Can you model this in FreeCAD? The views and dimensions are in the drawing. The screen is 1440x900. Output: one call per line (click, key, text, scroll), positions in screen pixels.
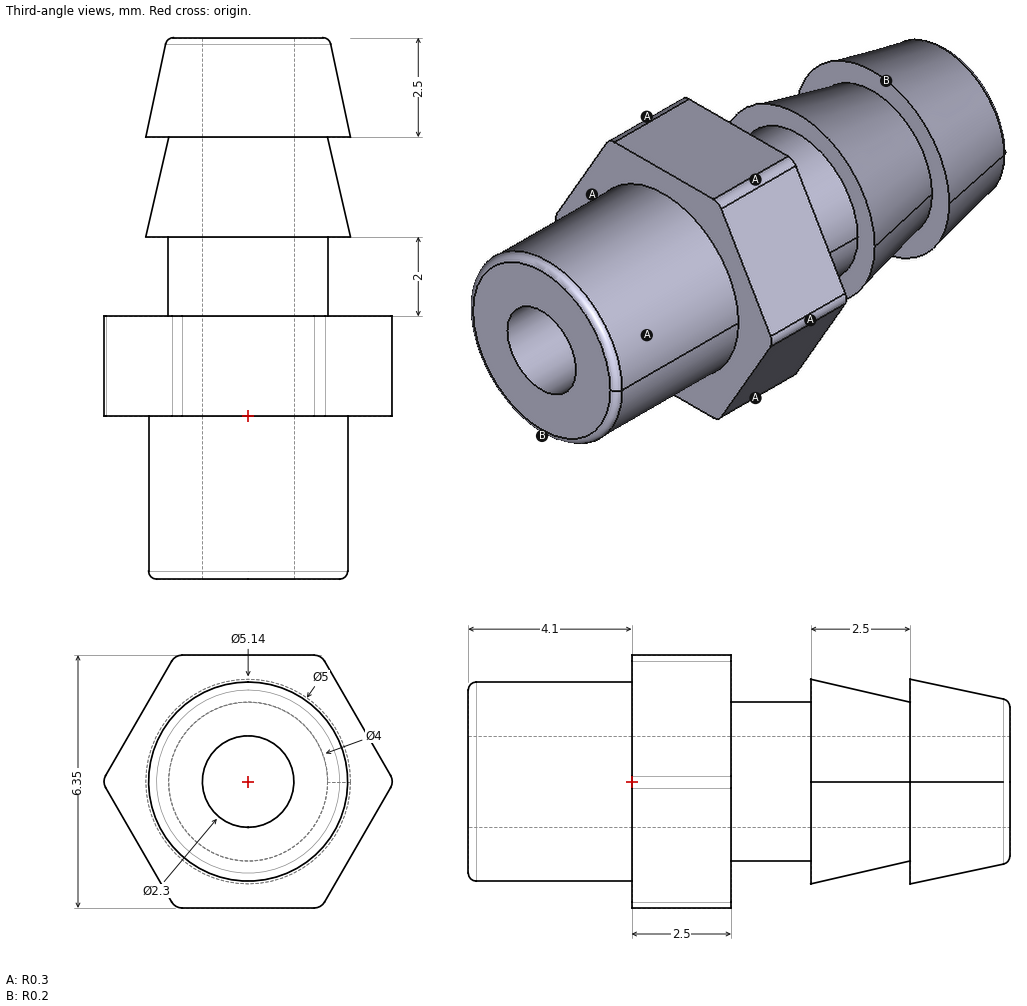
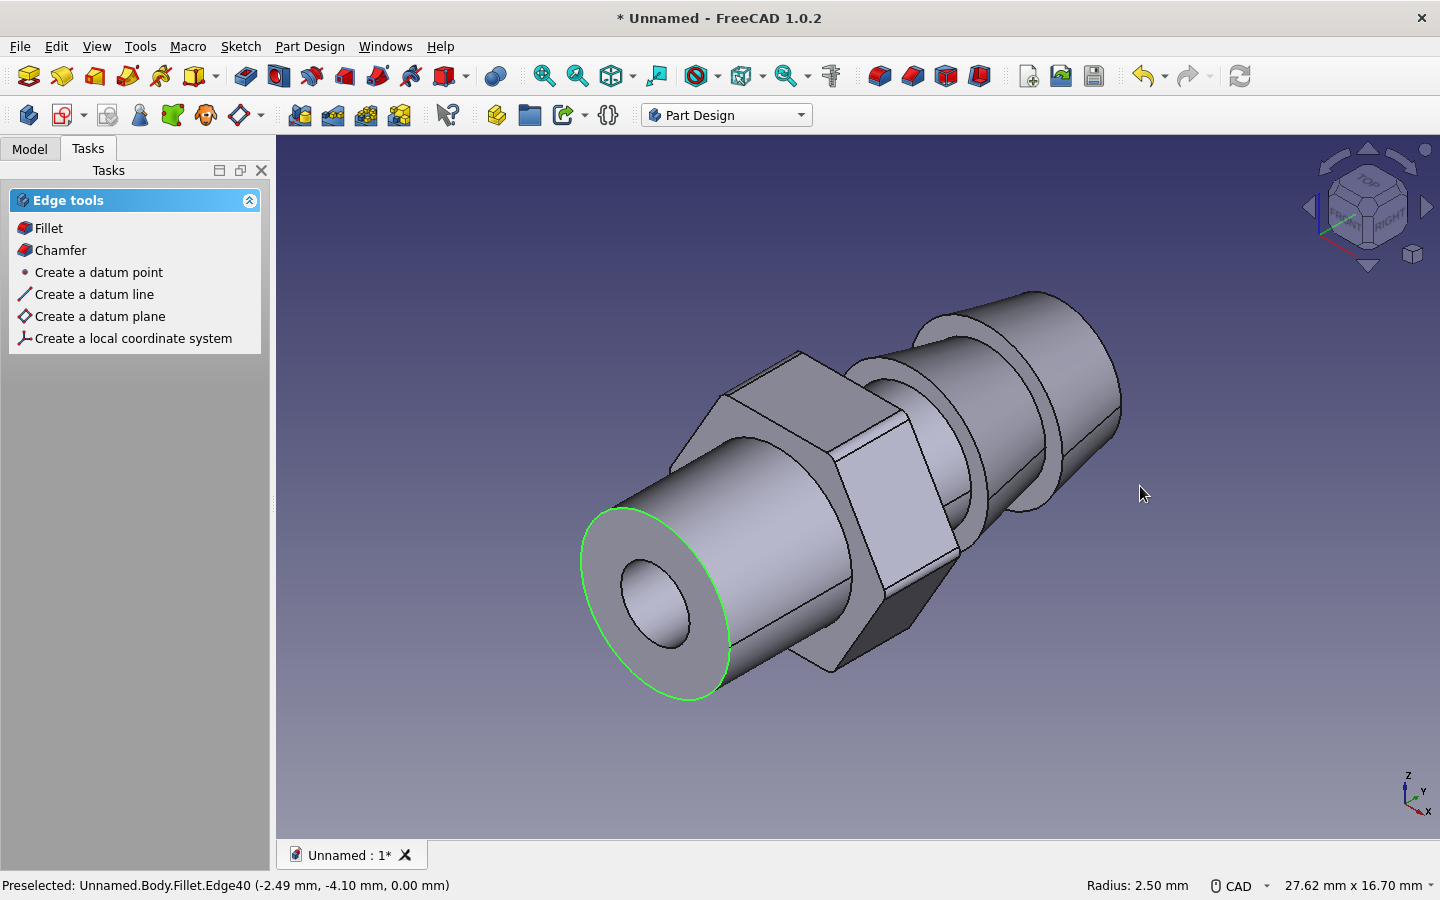
click(1042, 291, ctrl)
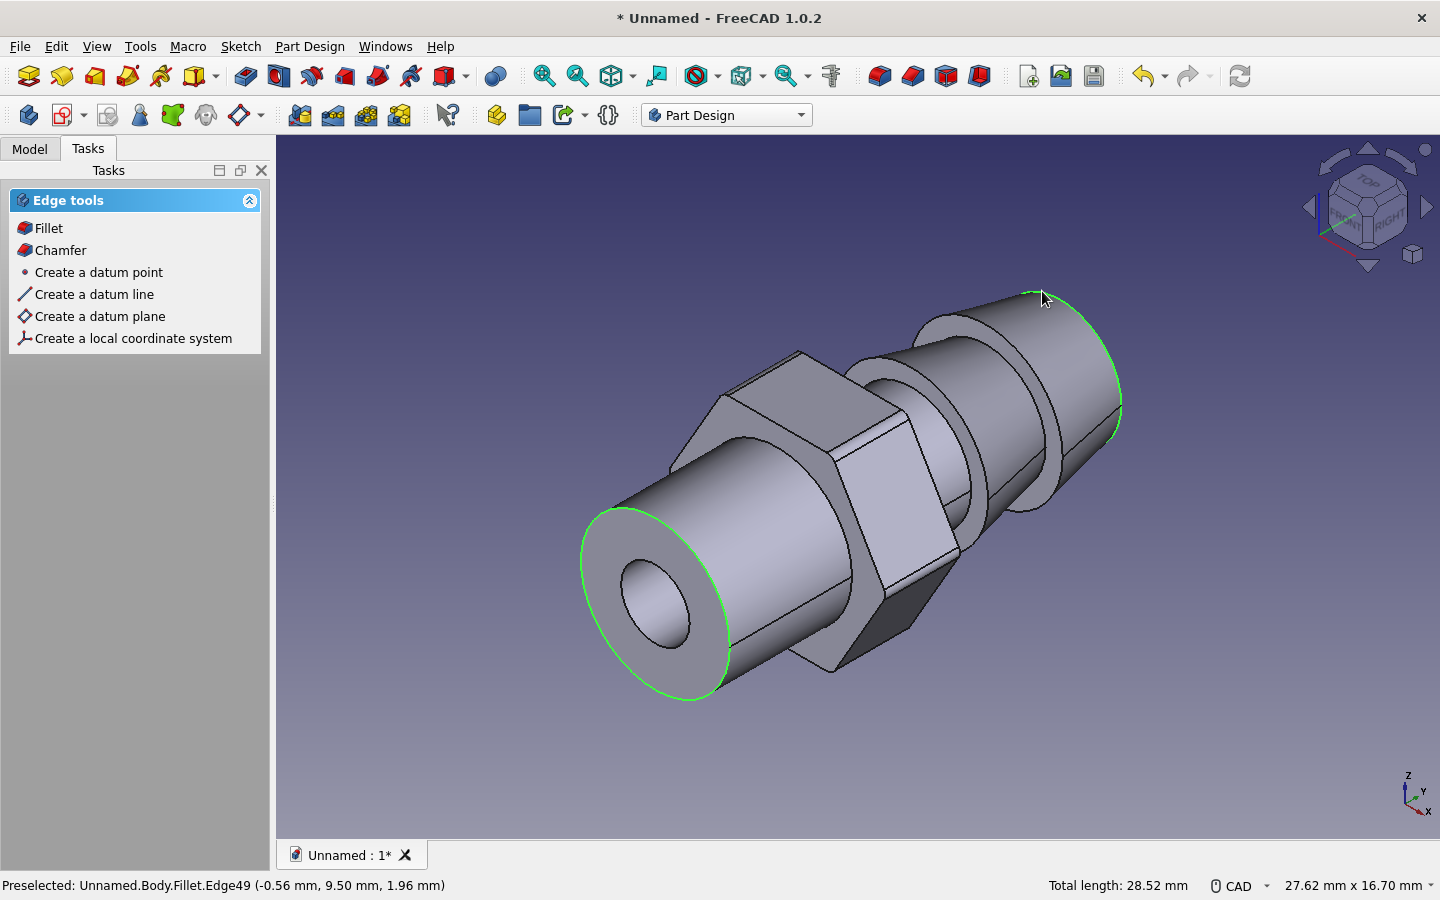
click(880, 76)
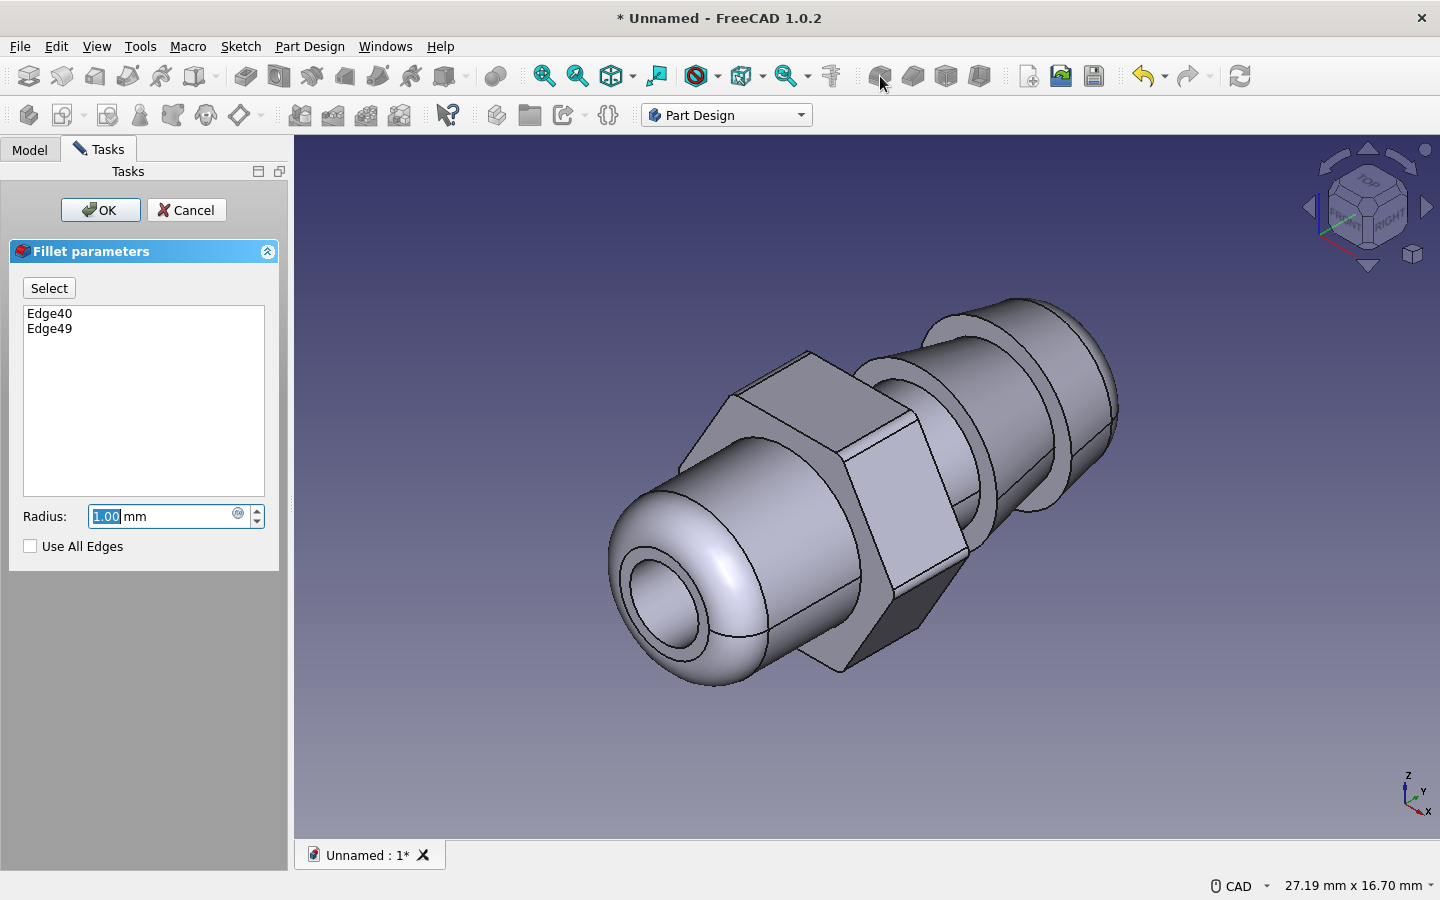
text(0.2)
key(Tab)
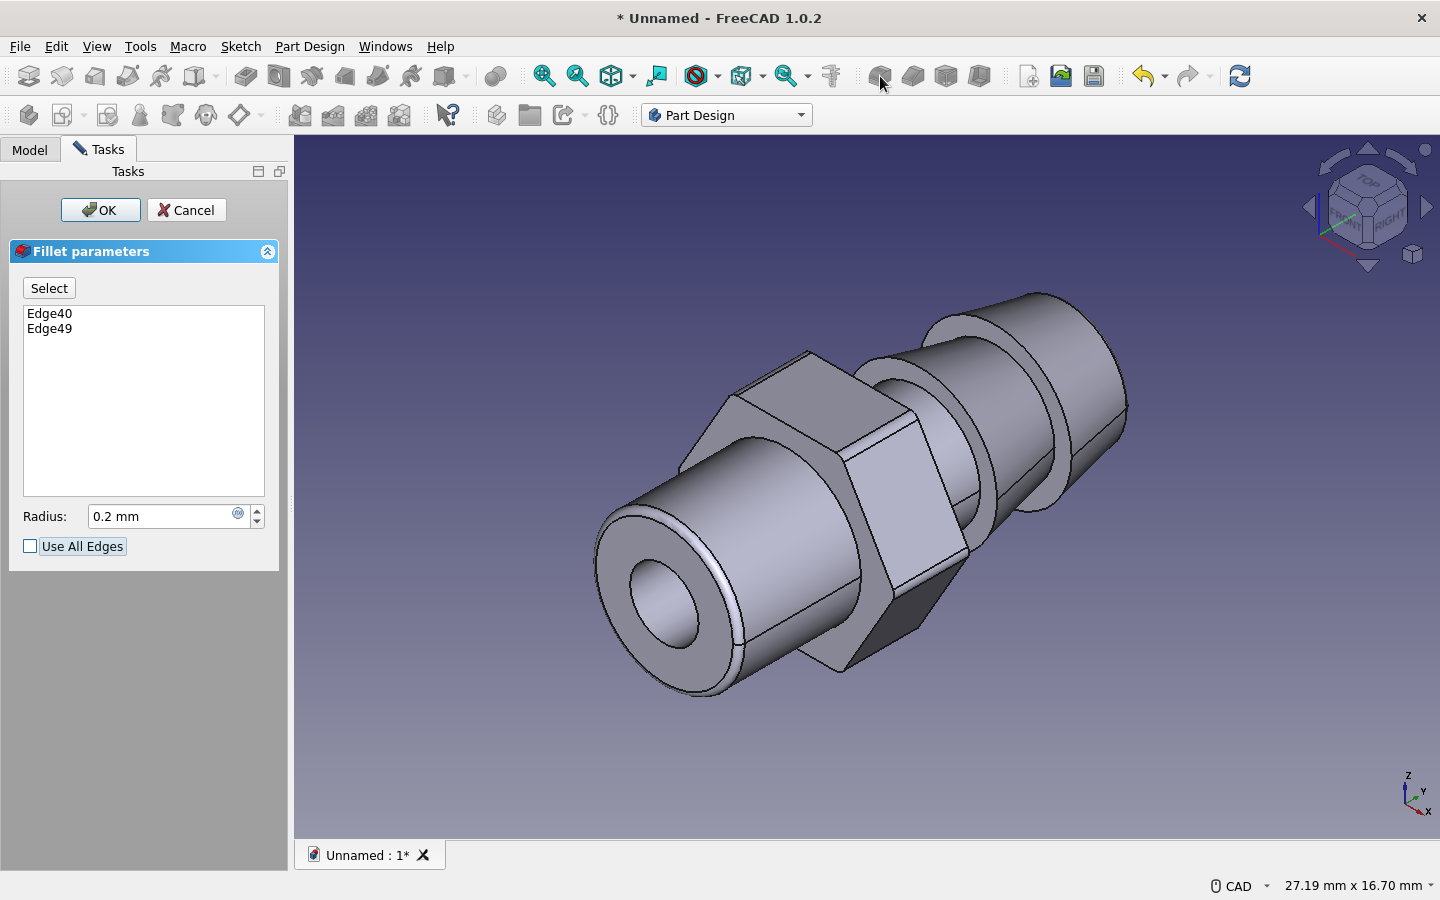
click(101, 210)